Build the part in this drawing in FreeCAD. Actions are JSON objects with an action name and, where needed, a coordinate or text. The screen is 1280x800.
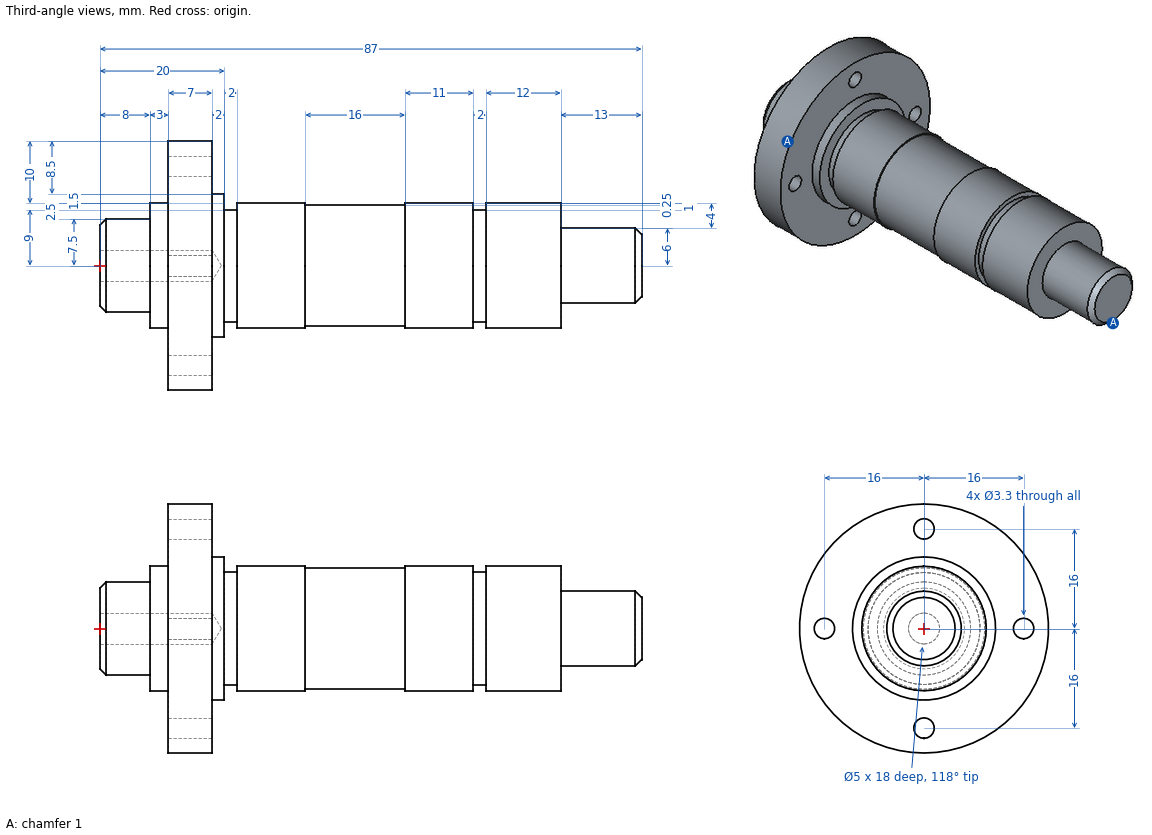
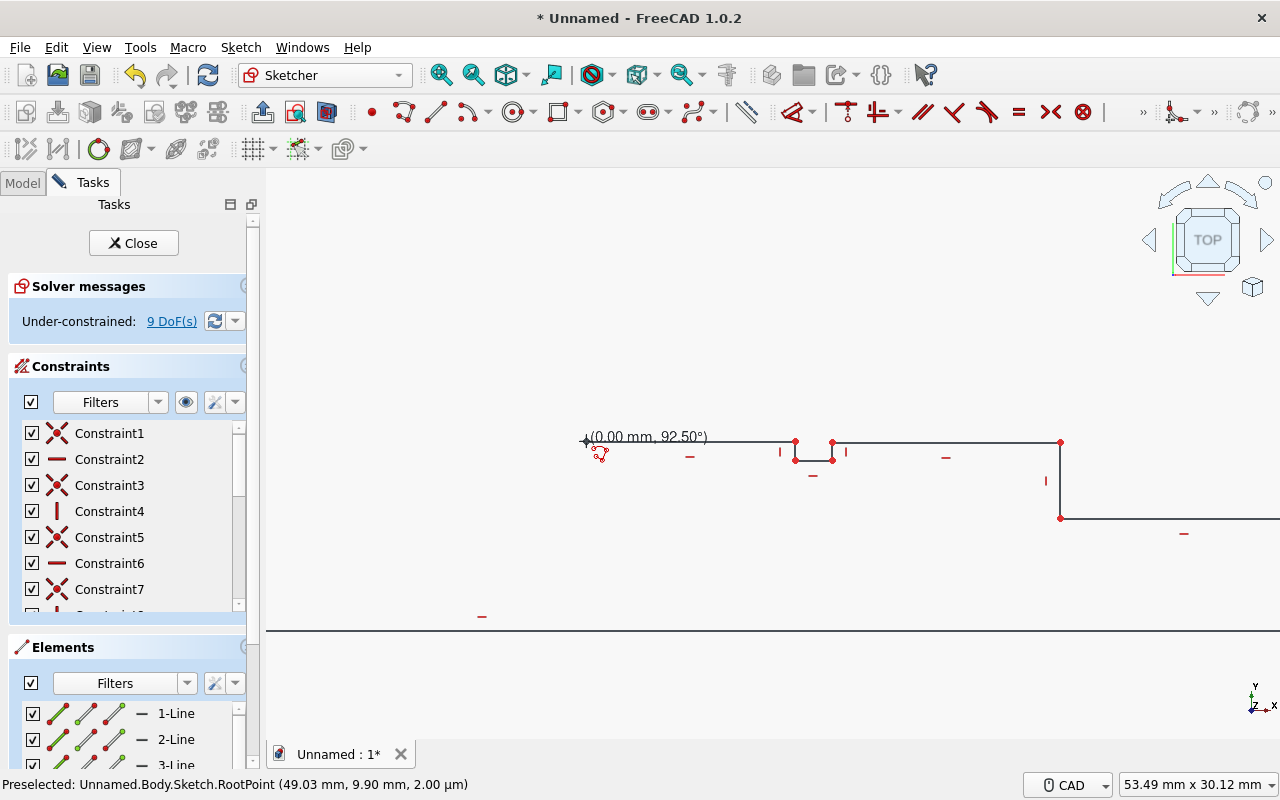
{"action": "scroll", "coordinate": [586, 446], "scroll_direction": "up", "scroll_amount": 7}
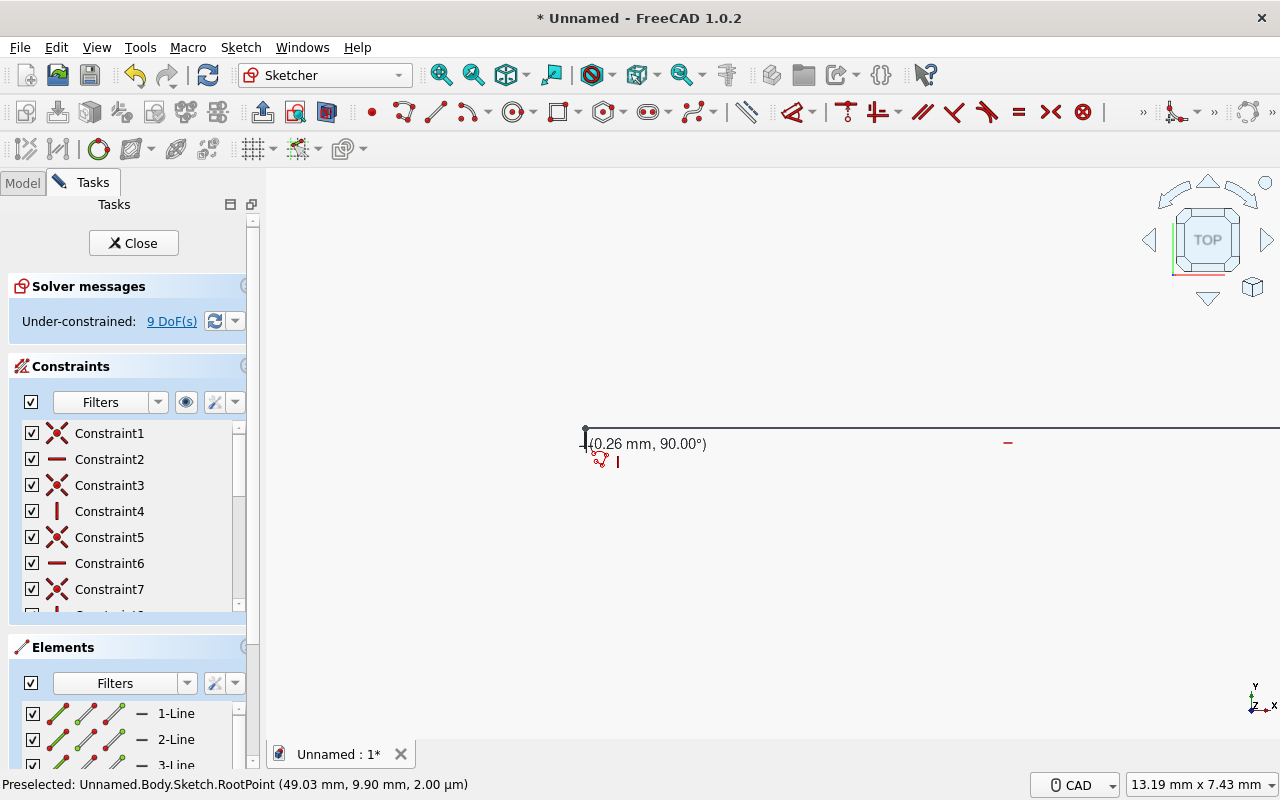
{"action": "left_click", "coordinate": [585, 444]}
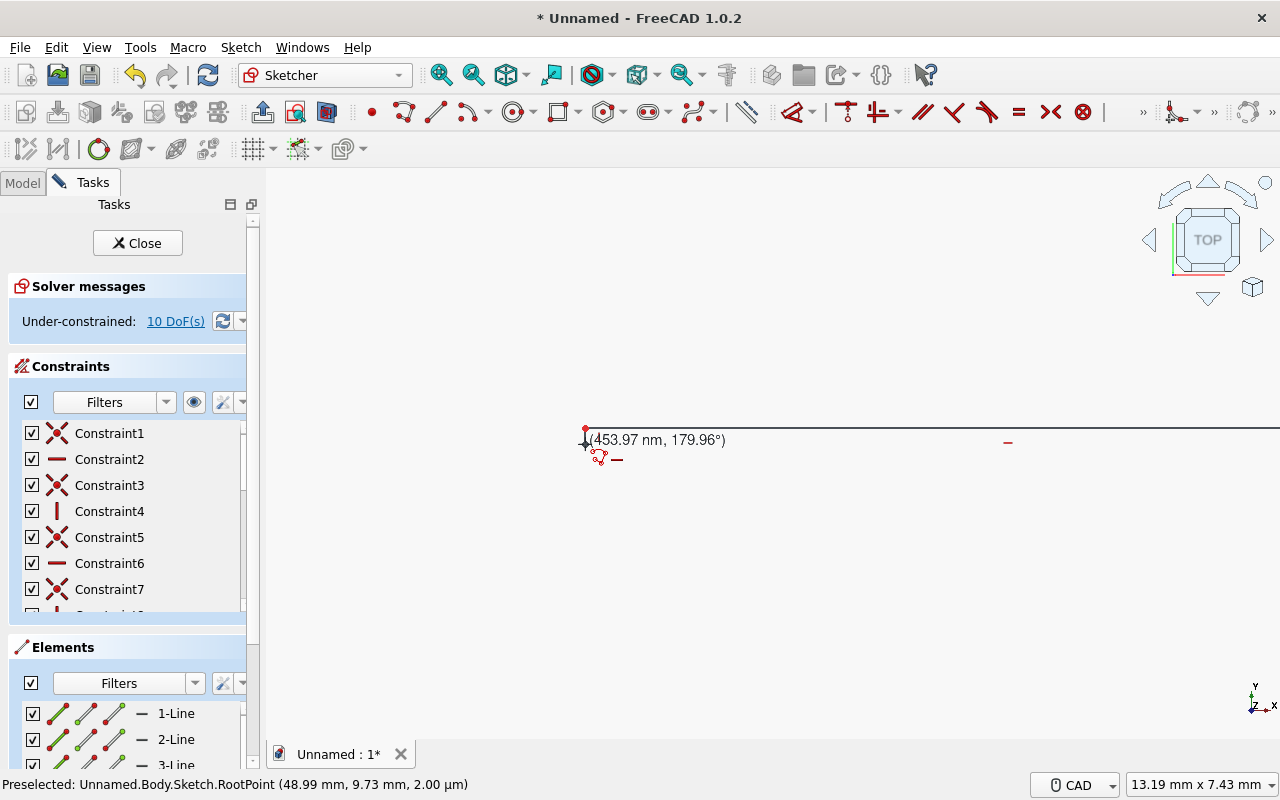
{"action": "scroll", "coordinate": [758, 456], "scroll_direction": "down", "scroll_amount": 12}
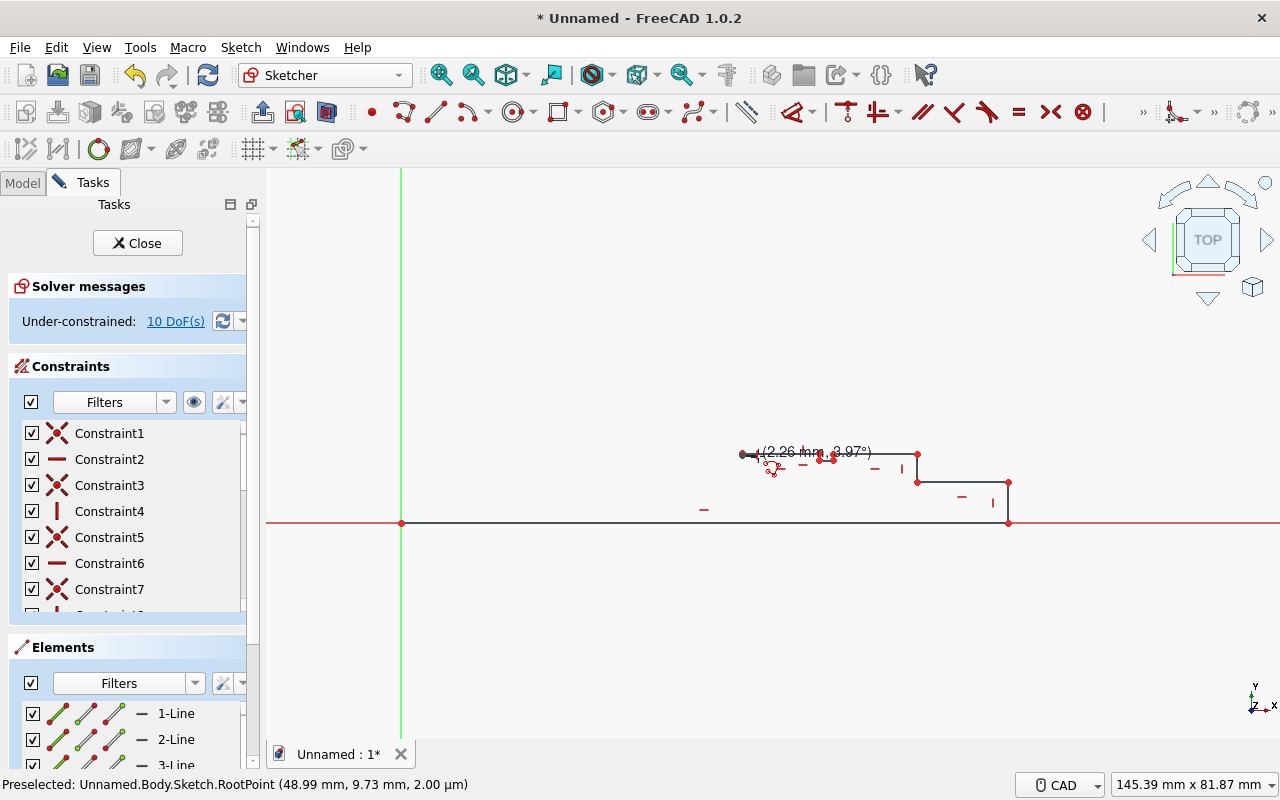
{"action": "left_click", "coordinate": [631, 455]}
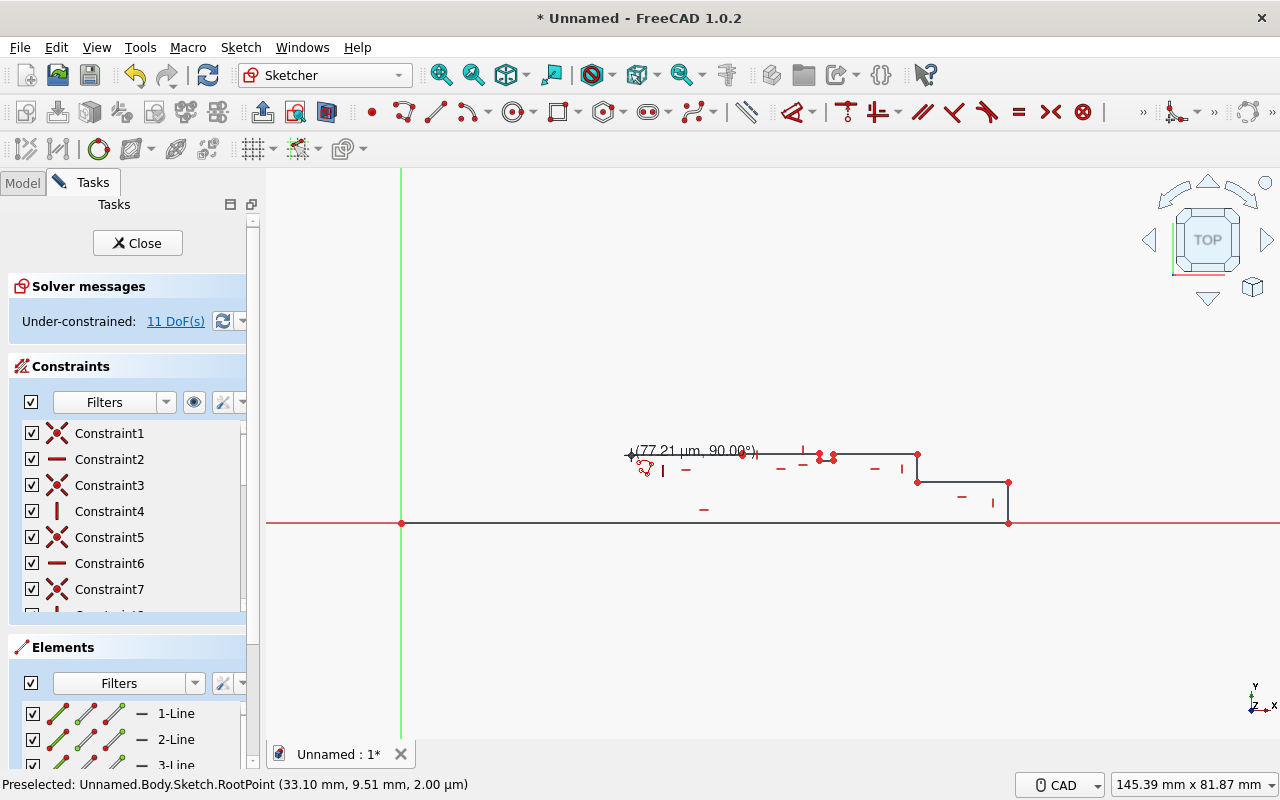
{"action": "scroll", "coordinate": [631, 454], "scroll_direction": "up", "scroll_amount": 12}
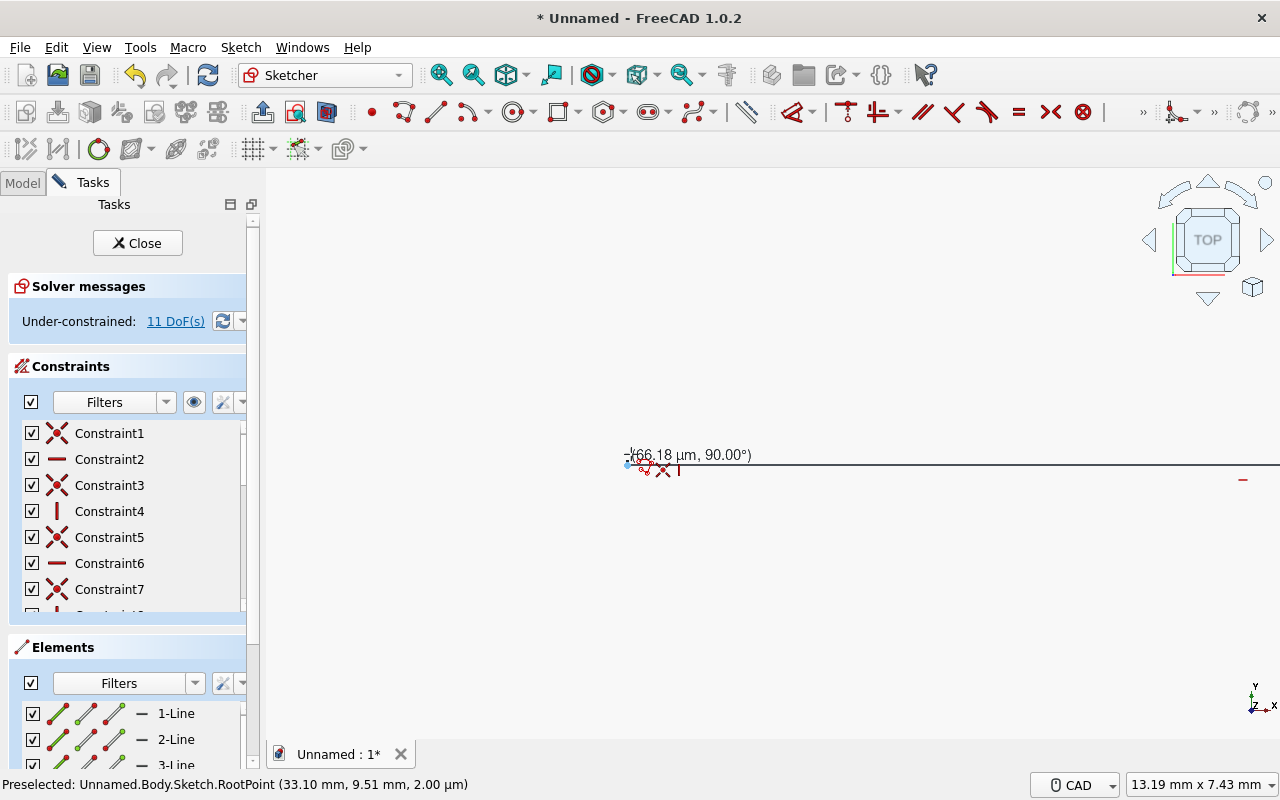
{"action": "left_click", "coordinate": [627, 444]}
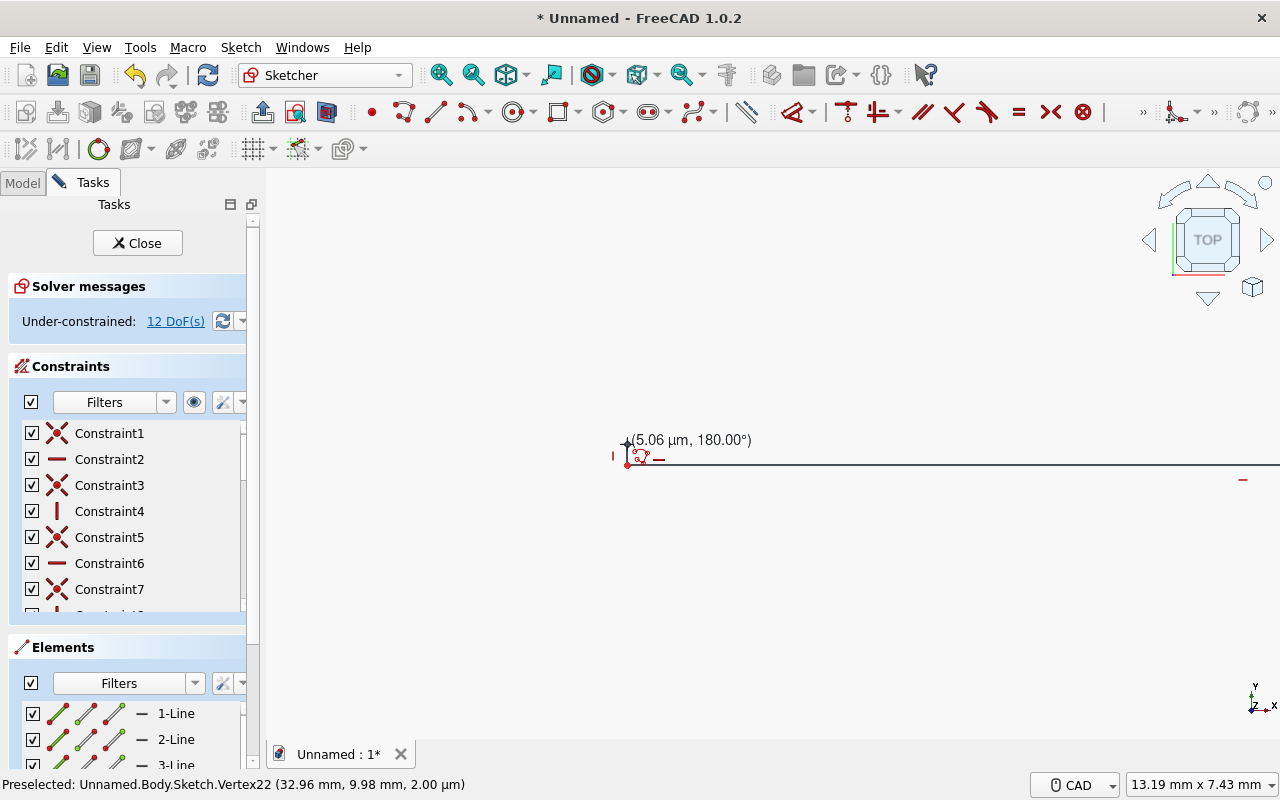
{"action": "scroll", "coordinate": [631, 454], "scroll_direction": "down", "scroll_amount": 12}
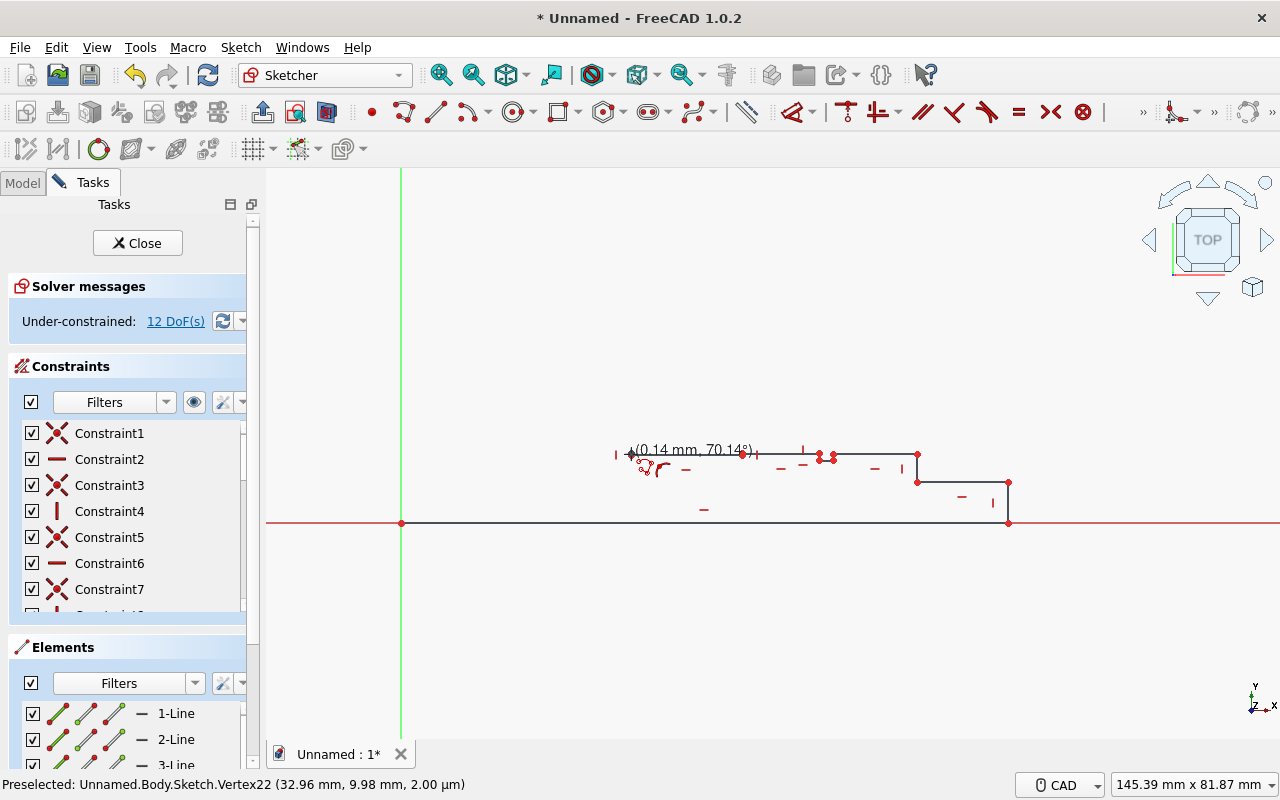
{"action": "left_click", "coordinate": [541, 454]}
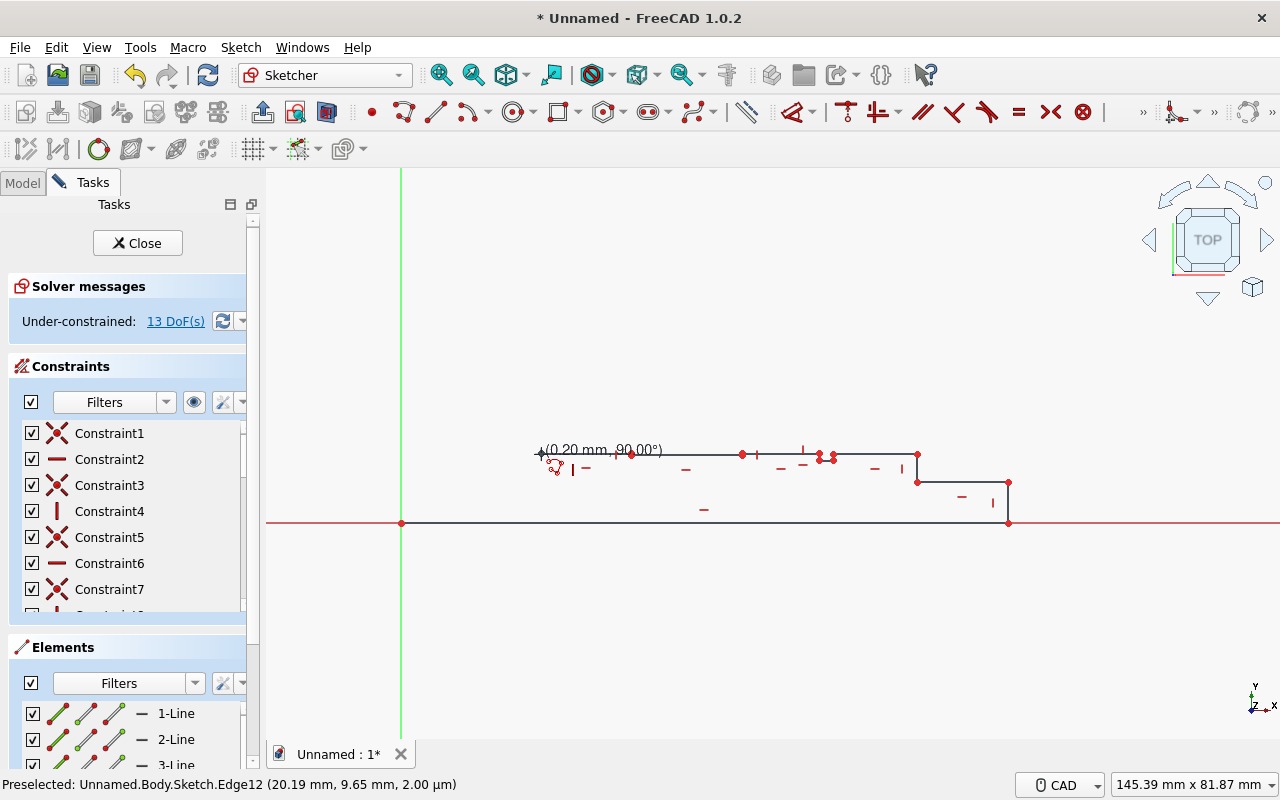
{"action": "scroll", "coordinate": [541, 443], "scroll_direction": "up", "scroll_amount": 3}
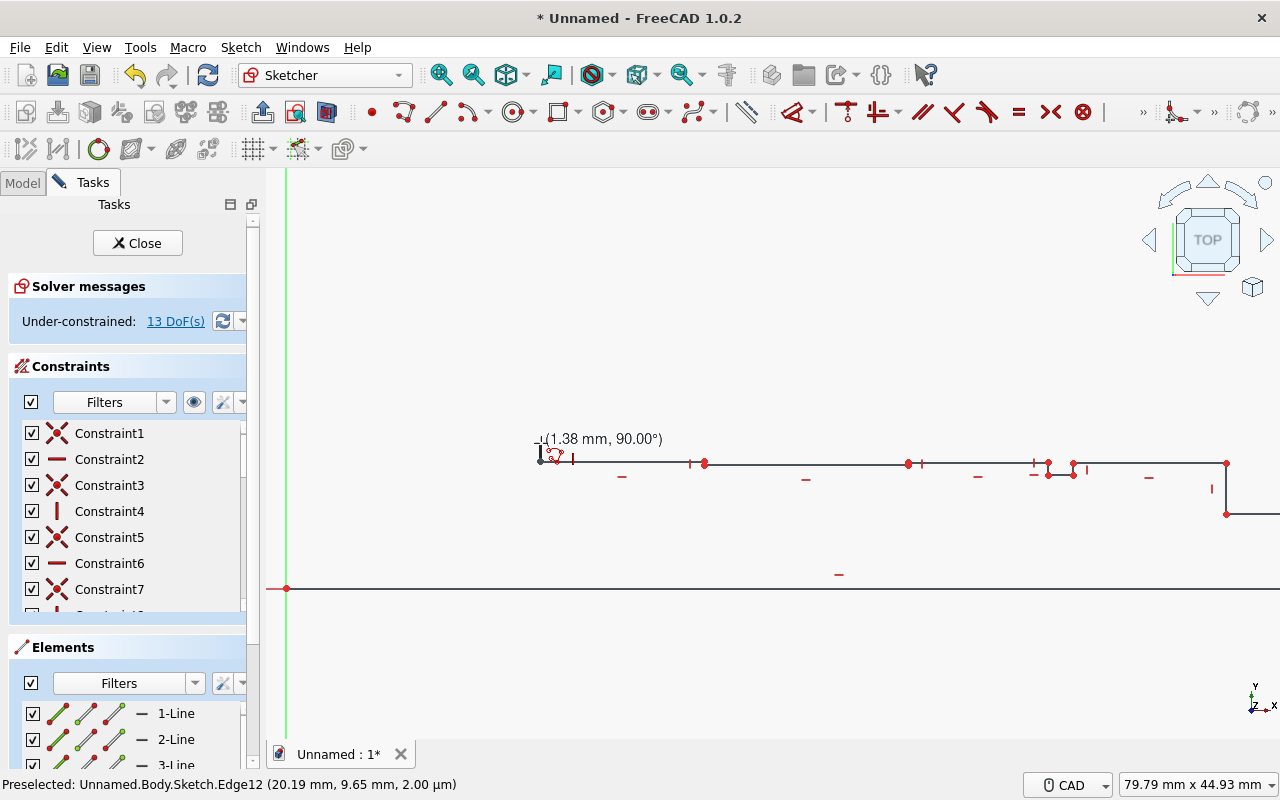
{"action": "left_click", "coordinate": [541, 443]}
{"action": "left_click", "coordinate": [515, 443]}
{"action": "left_click", "coordinate": [515, 335]}
{"action": "left_click", "coordinate": [426, 335]}
{"action": "left_click", "coordinate": [426, 462]}
{"action": "left_click", "coordinate": [388, 462]}
{"action": "left_click", "coordinate": [388, 494]}